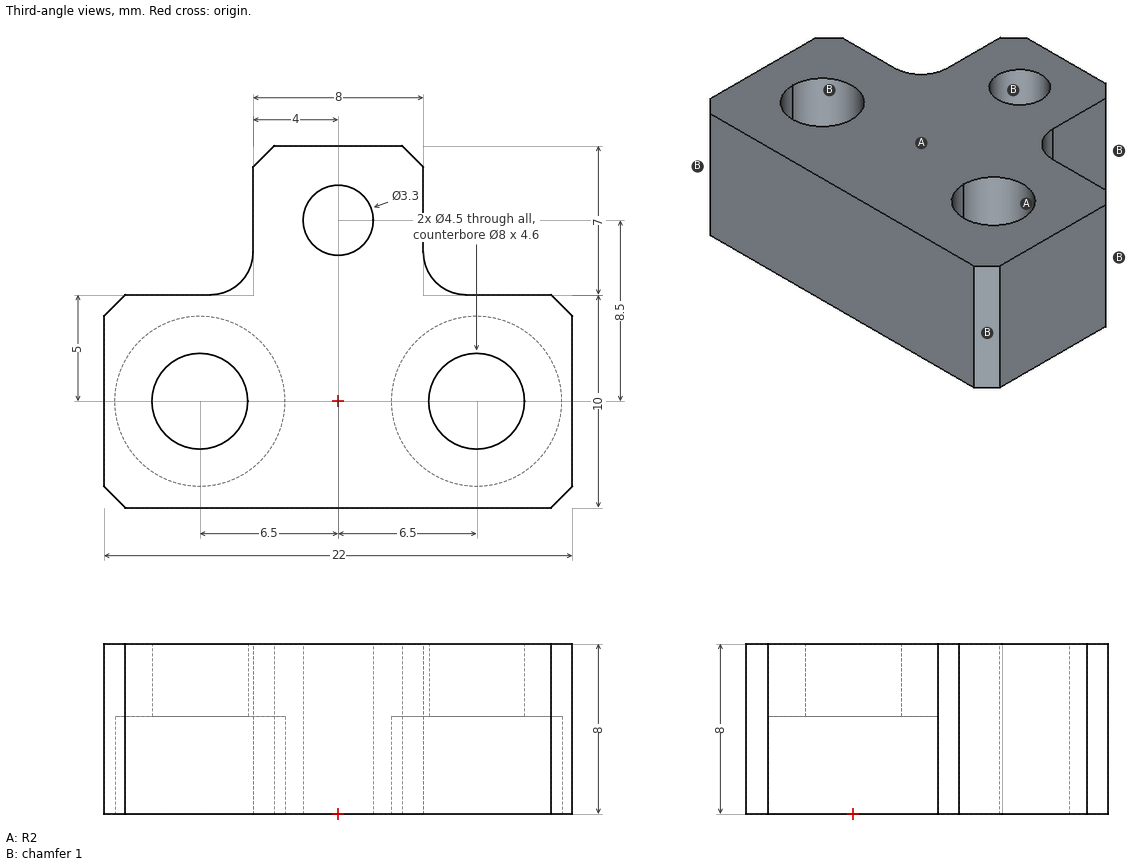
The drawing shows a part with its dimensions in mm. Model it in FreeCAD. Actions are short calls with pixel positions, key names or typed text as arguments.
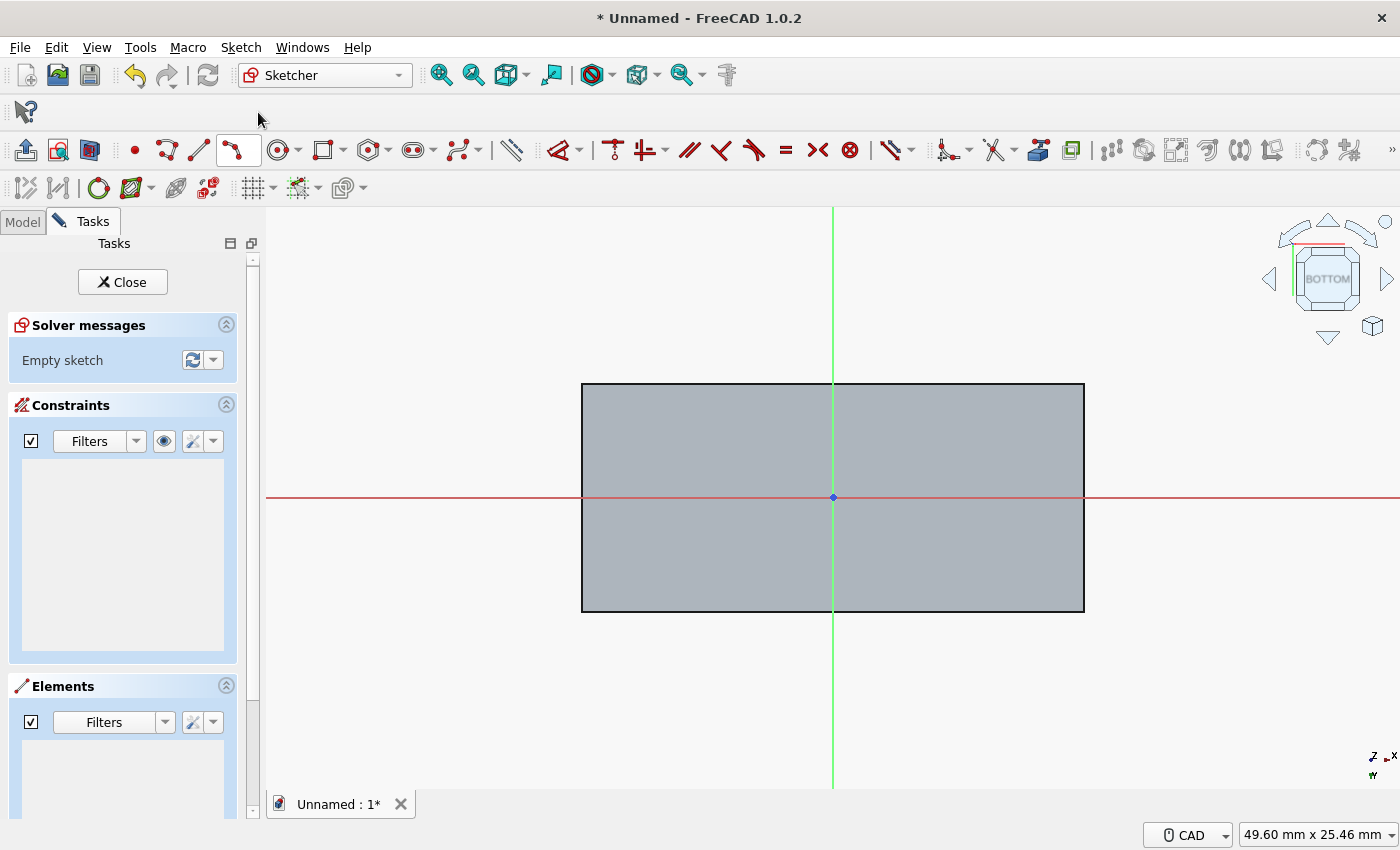
scroll(916, 498, up, 3)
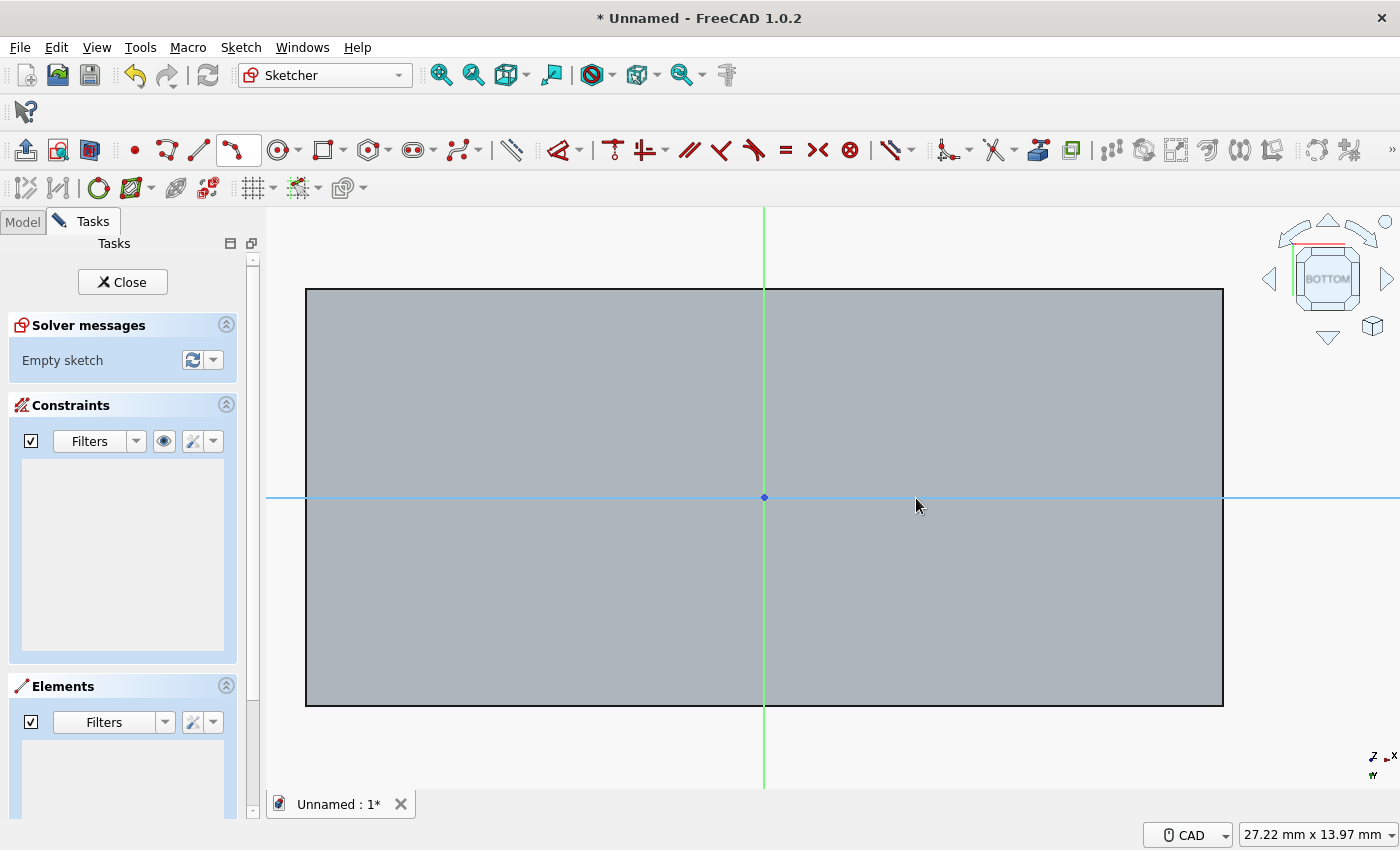
click(278, 150)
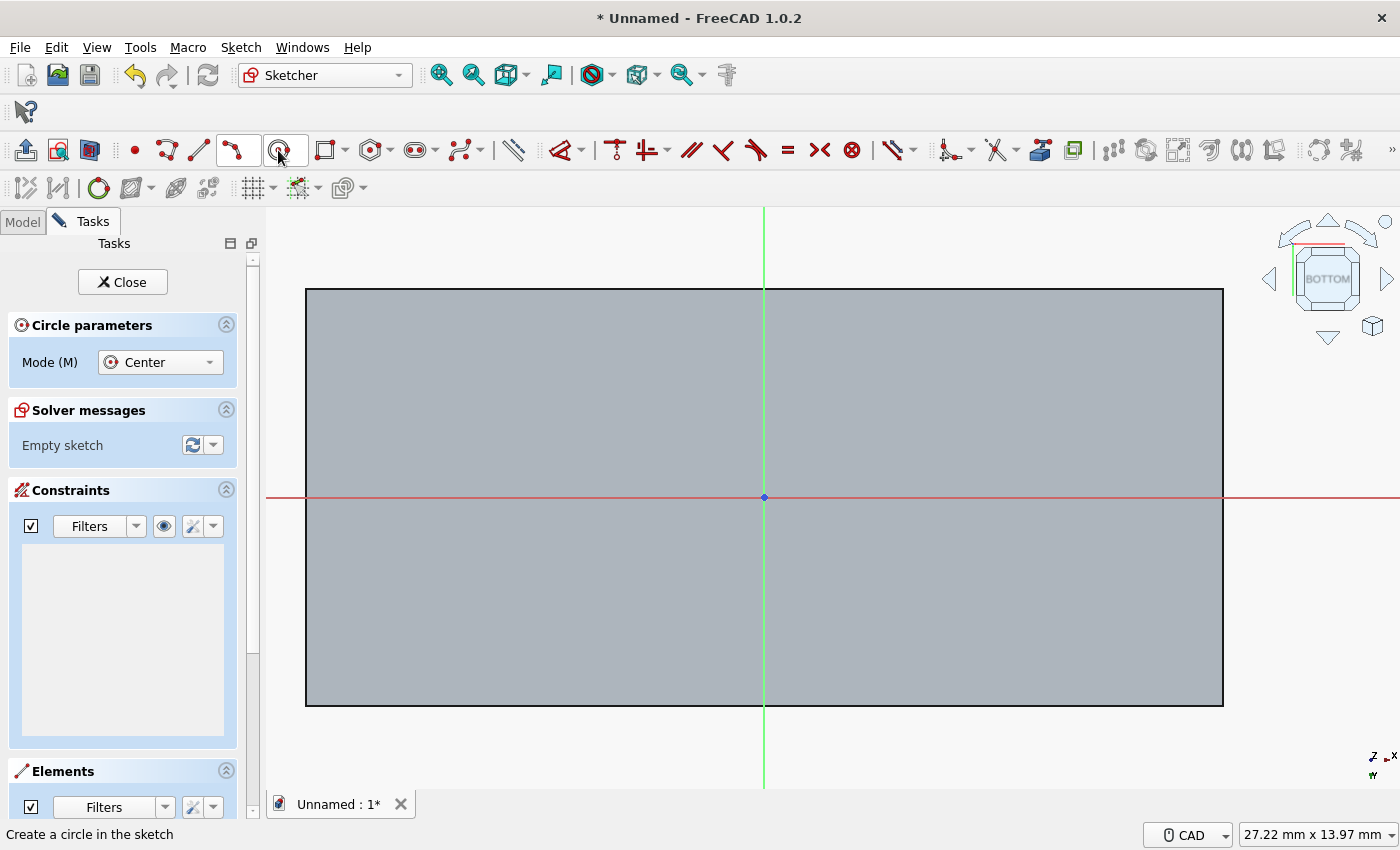
click(1035, 498)
move(1101, 431)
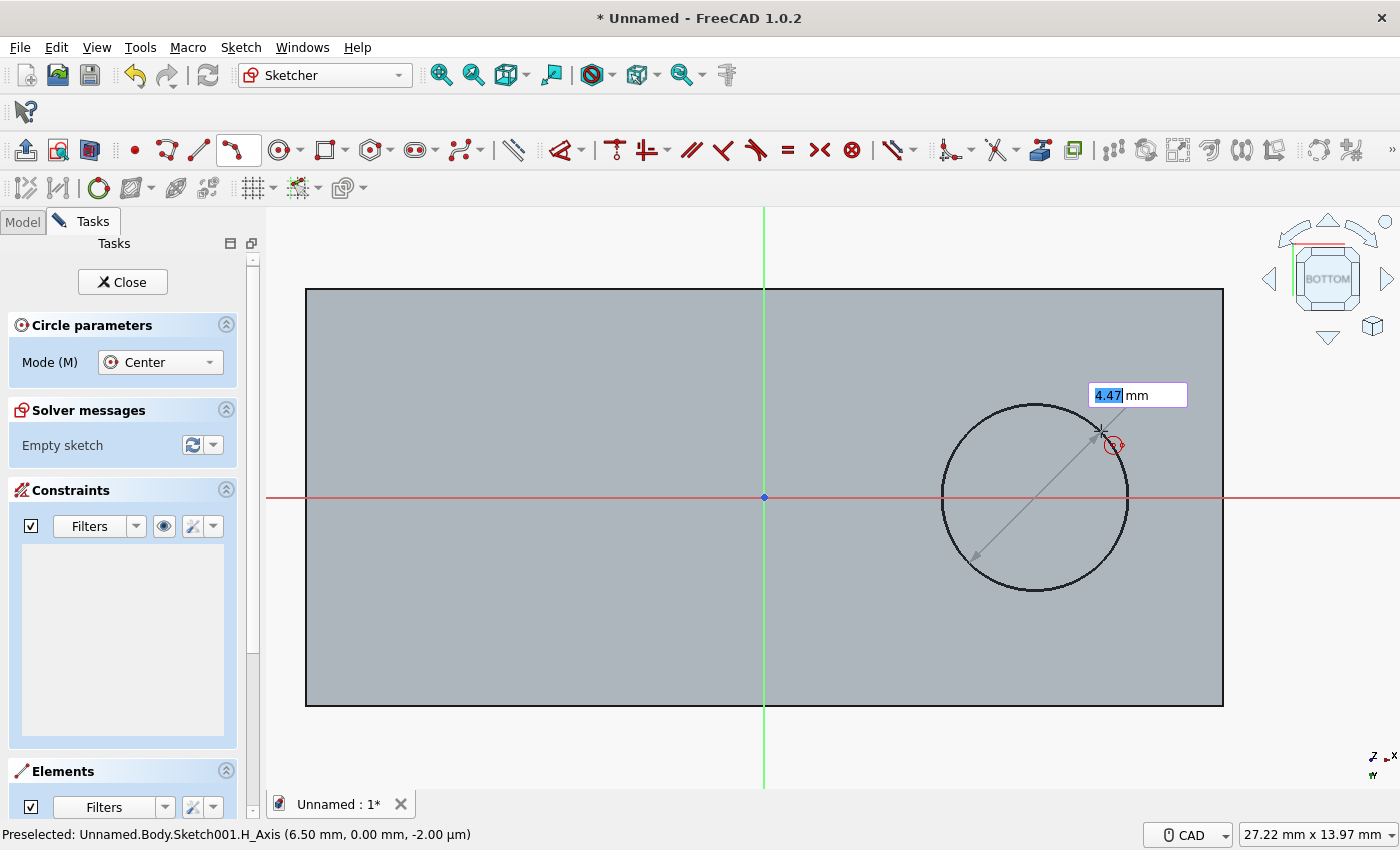
text(4.5)
key(Return)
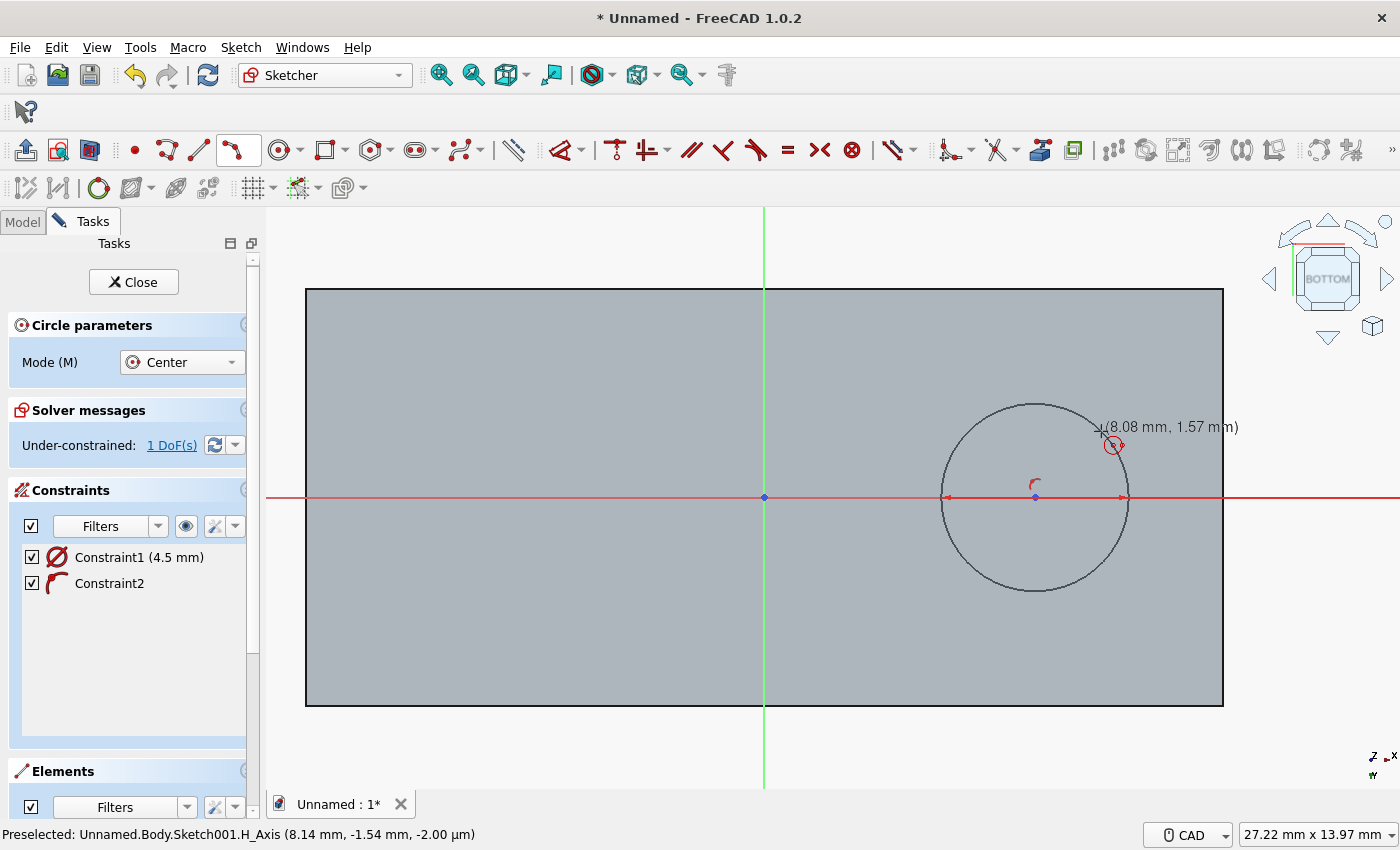
click(494, 498)
move(560, 431)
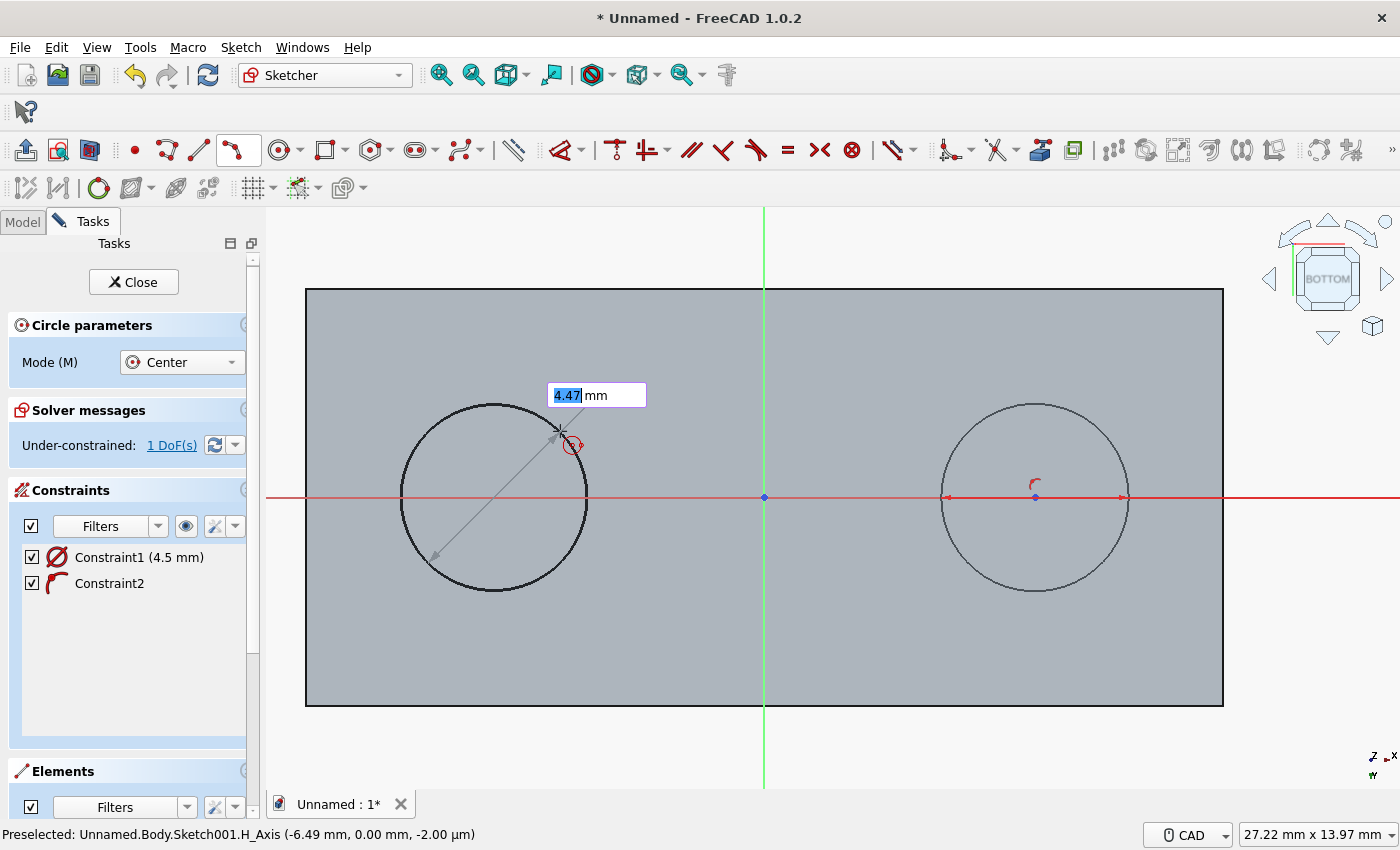
text(4.5)
key(Return)
key(Escape)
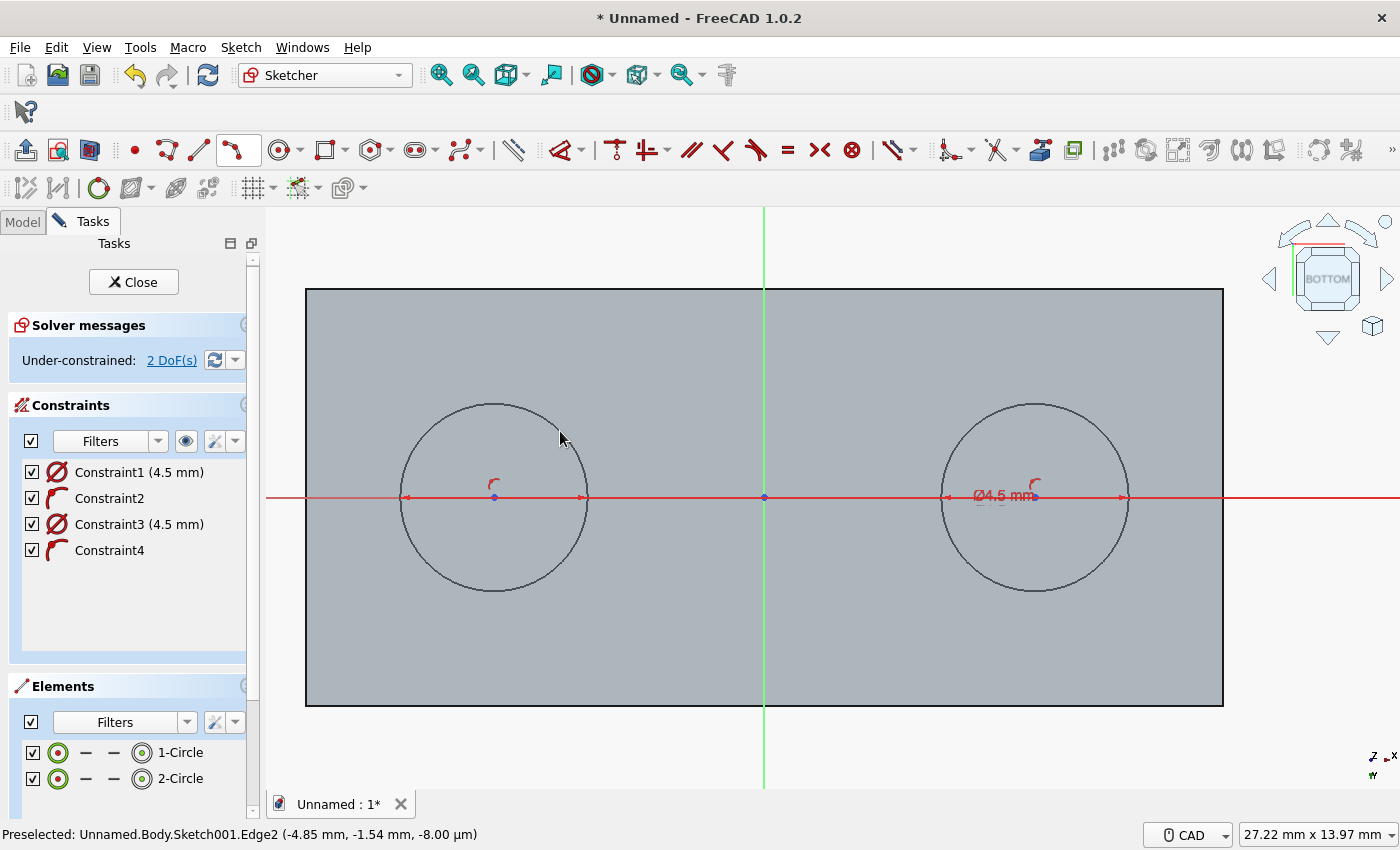
click(560, 150)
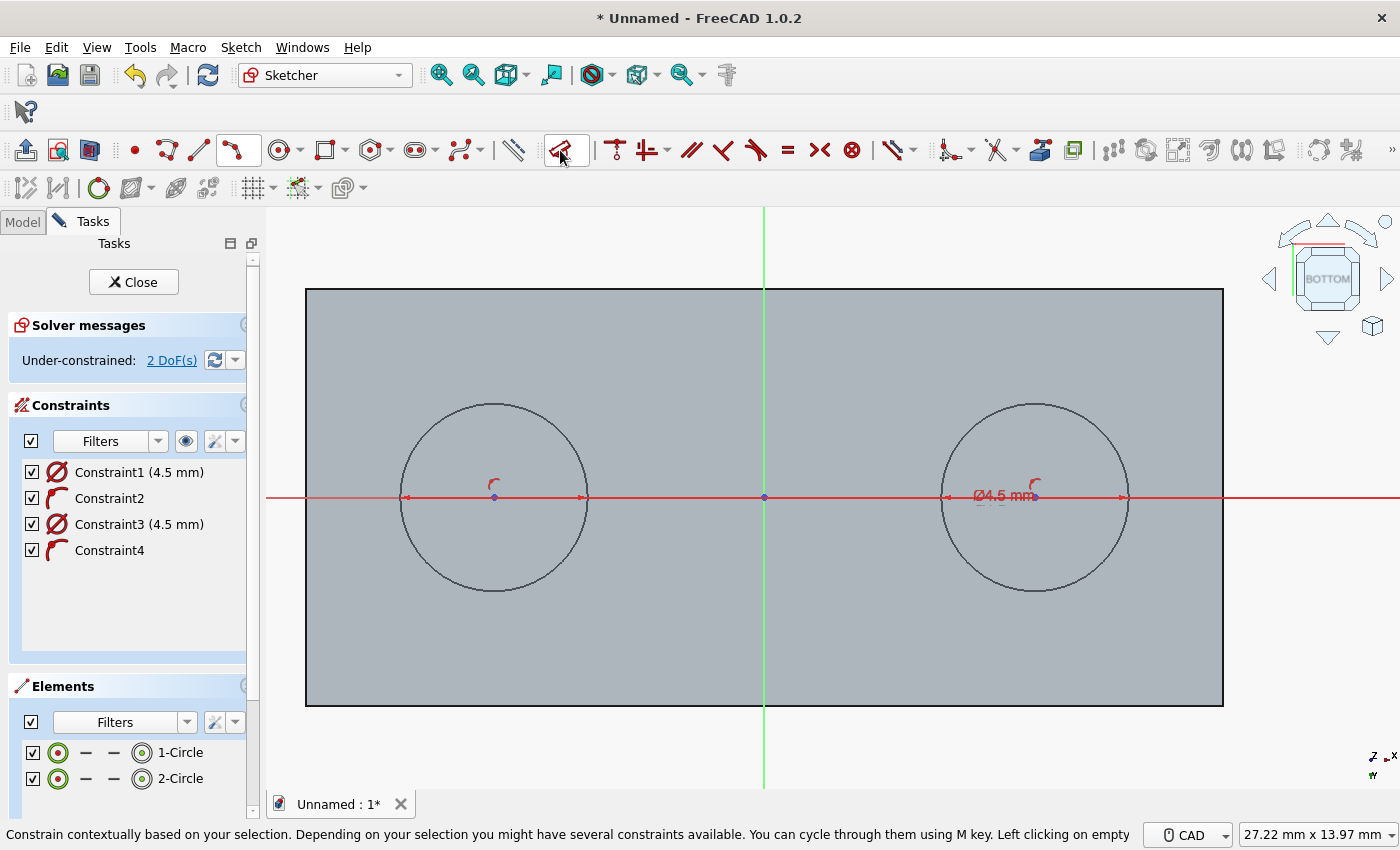
click(1035, 498)
click(900, 532)